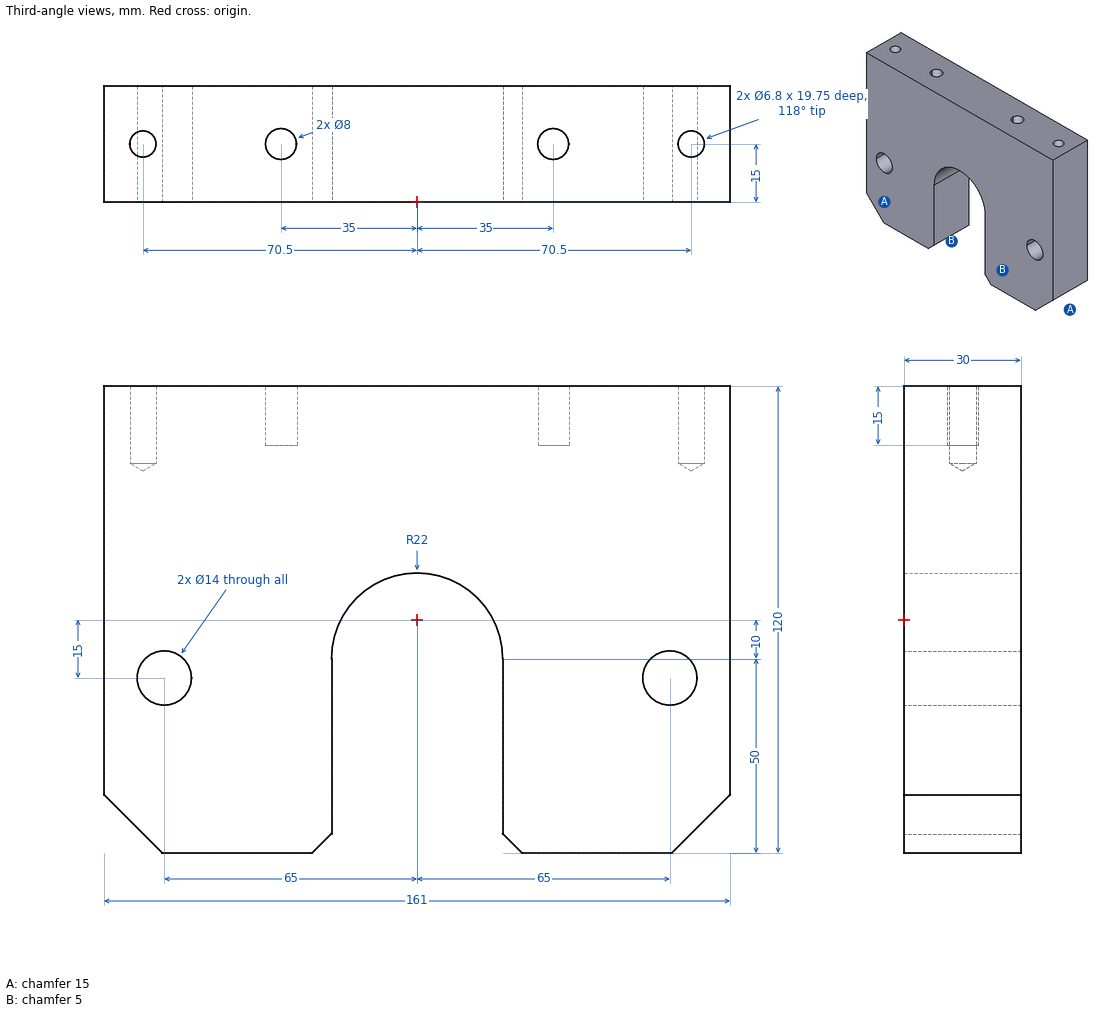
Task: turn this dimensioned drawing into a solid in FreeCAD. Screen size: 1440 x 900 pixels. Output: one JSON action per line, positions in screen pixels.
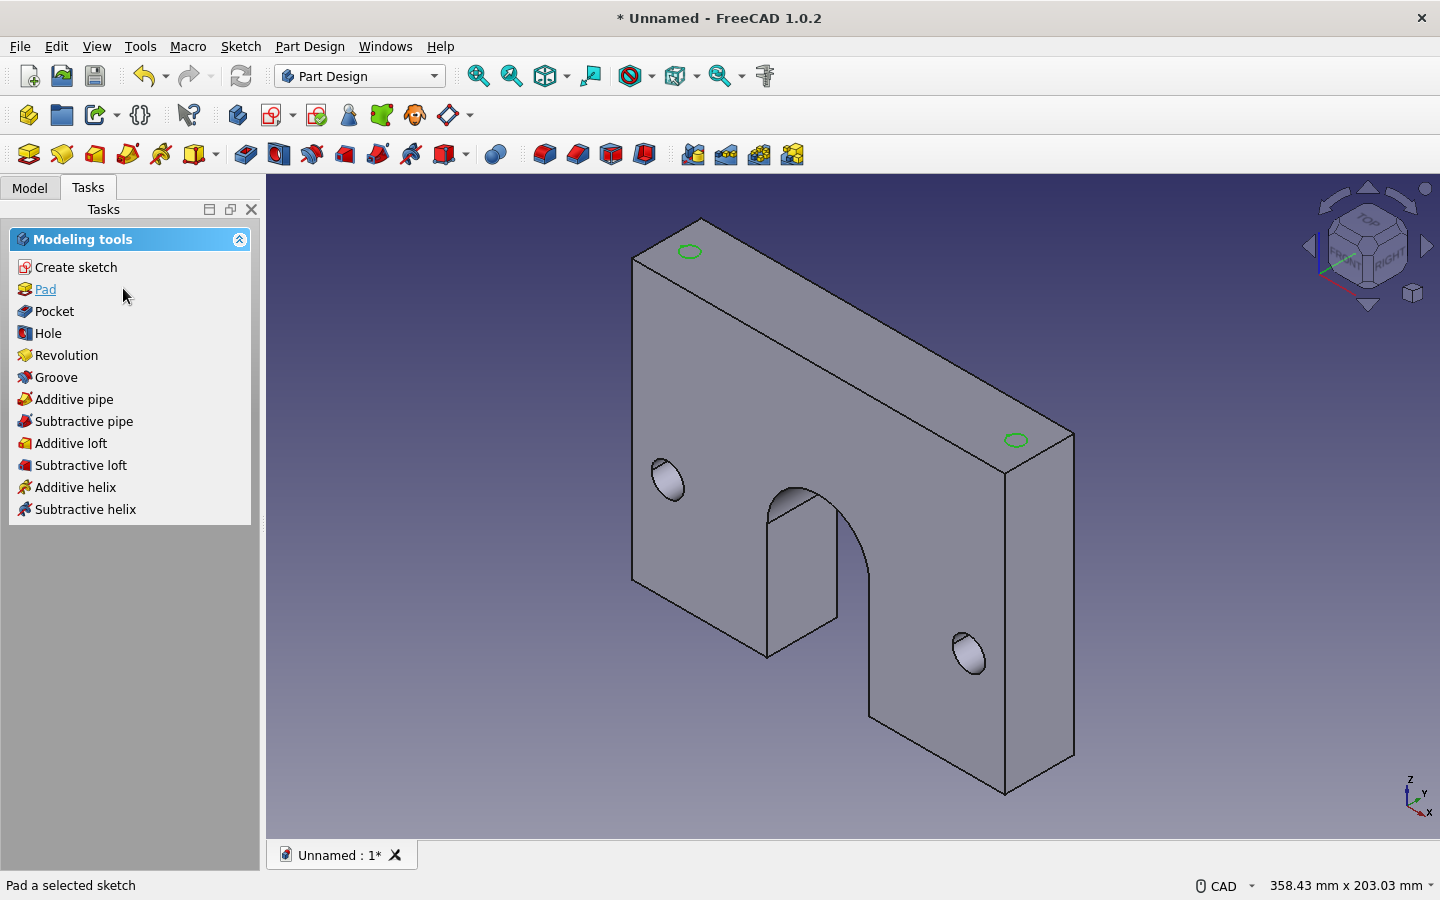
{"action": "left_click", "coordinate": [279, 154]}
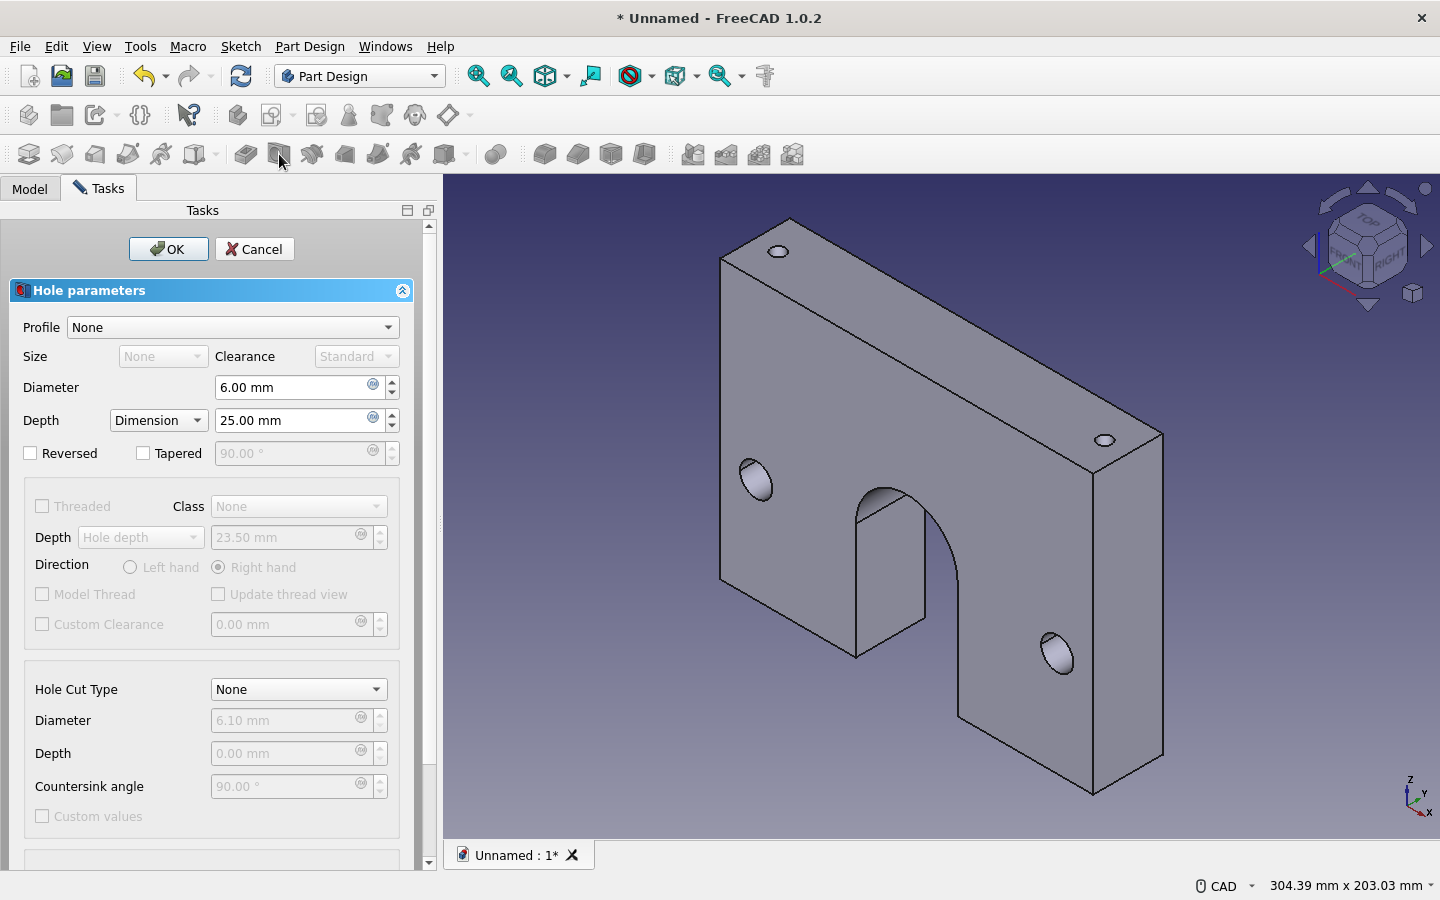
{"action": "triple_click", "coordinate": [300, 388]}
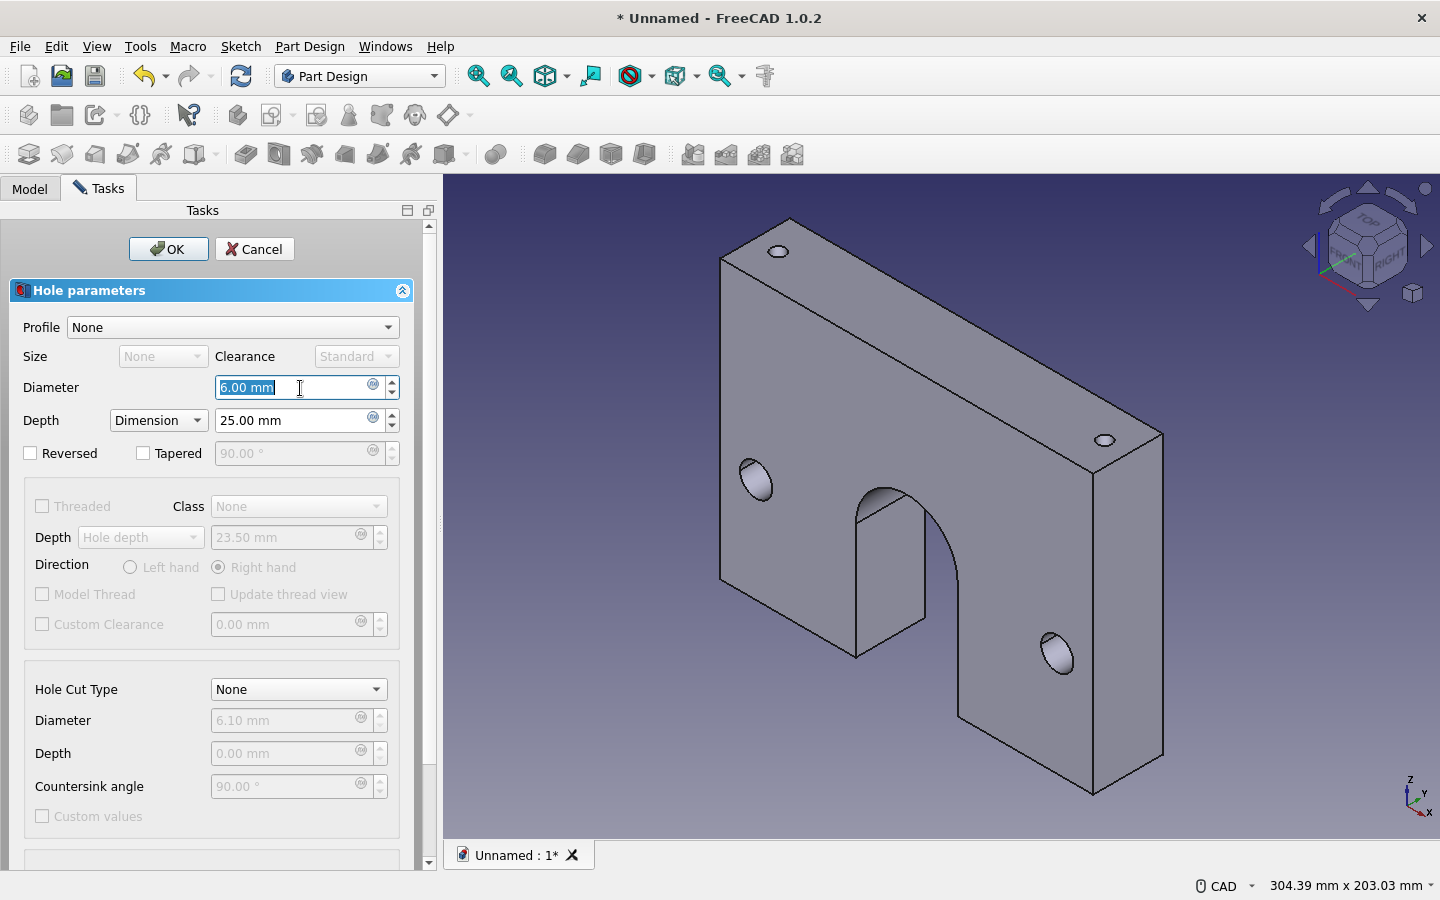
{"action": "type", "text": "6.8"}
{"action": "key", "text": "Tab"}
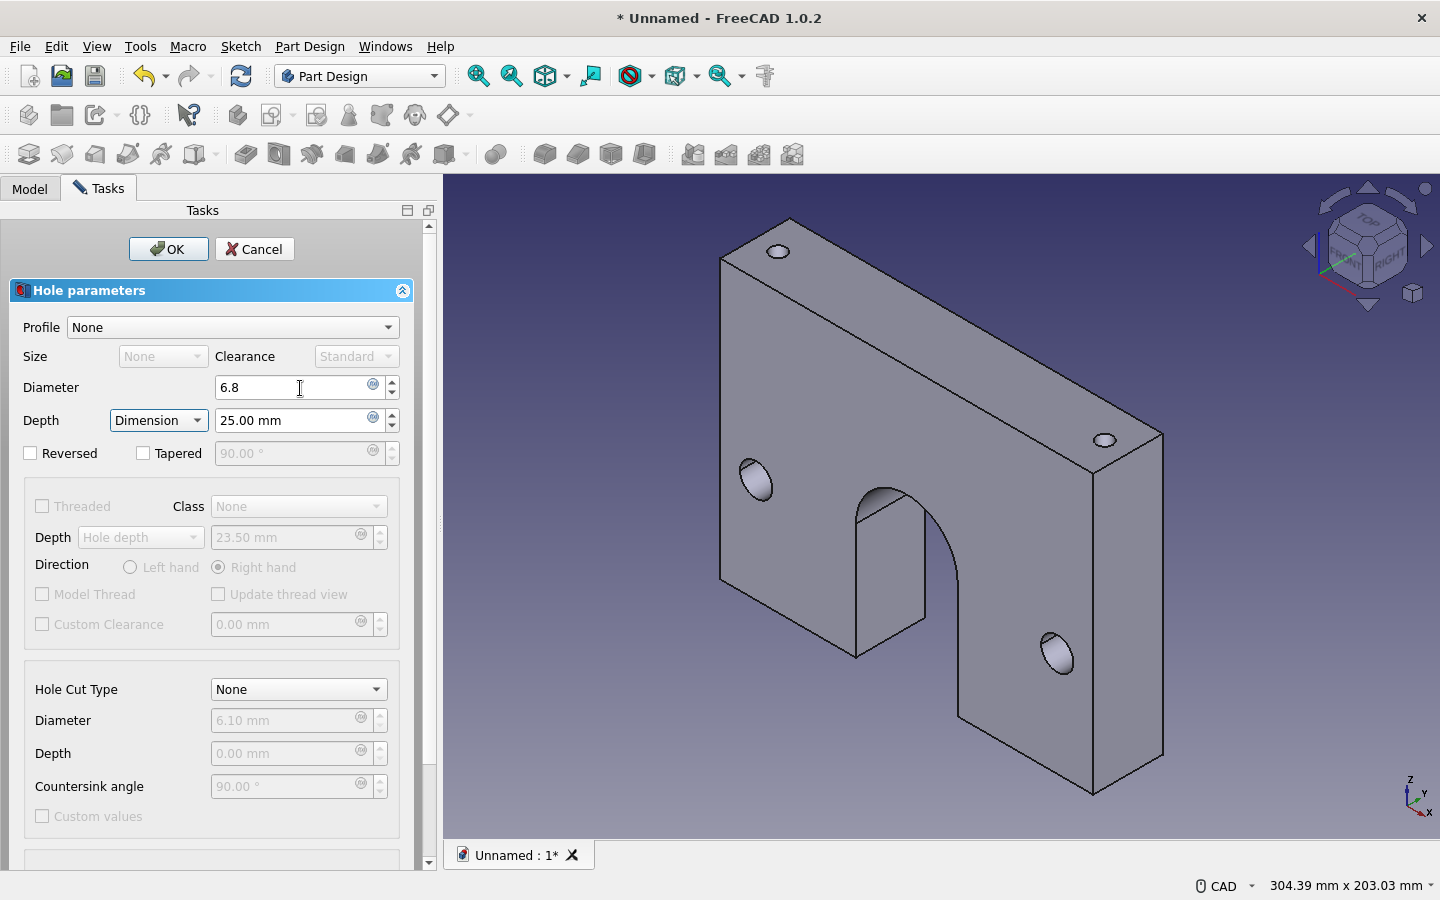
{"action": "triple_click", "coordinate": [300, 420]}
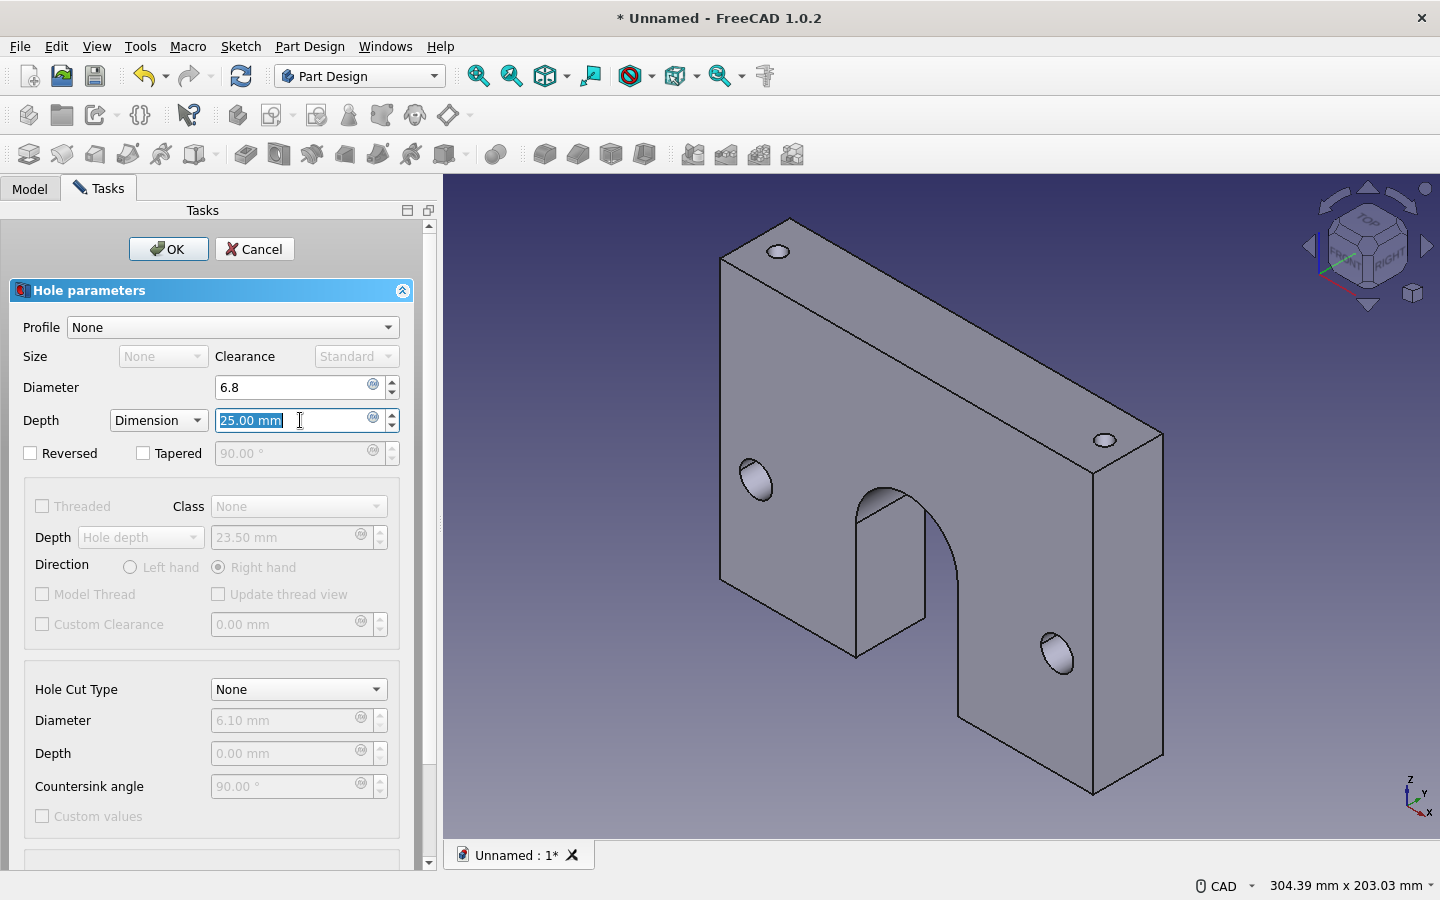
{"action": "type", "text": "19.75"}
{"action": "key", "text": "Tab"}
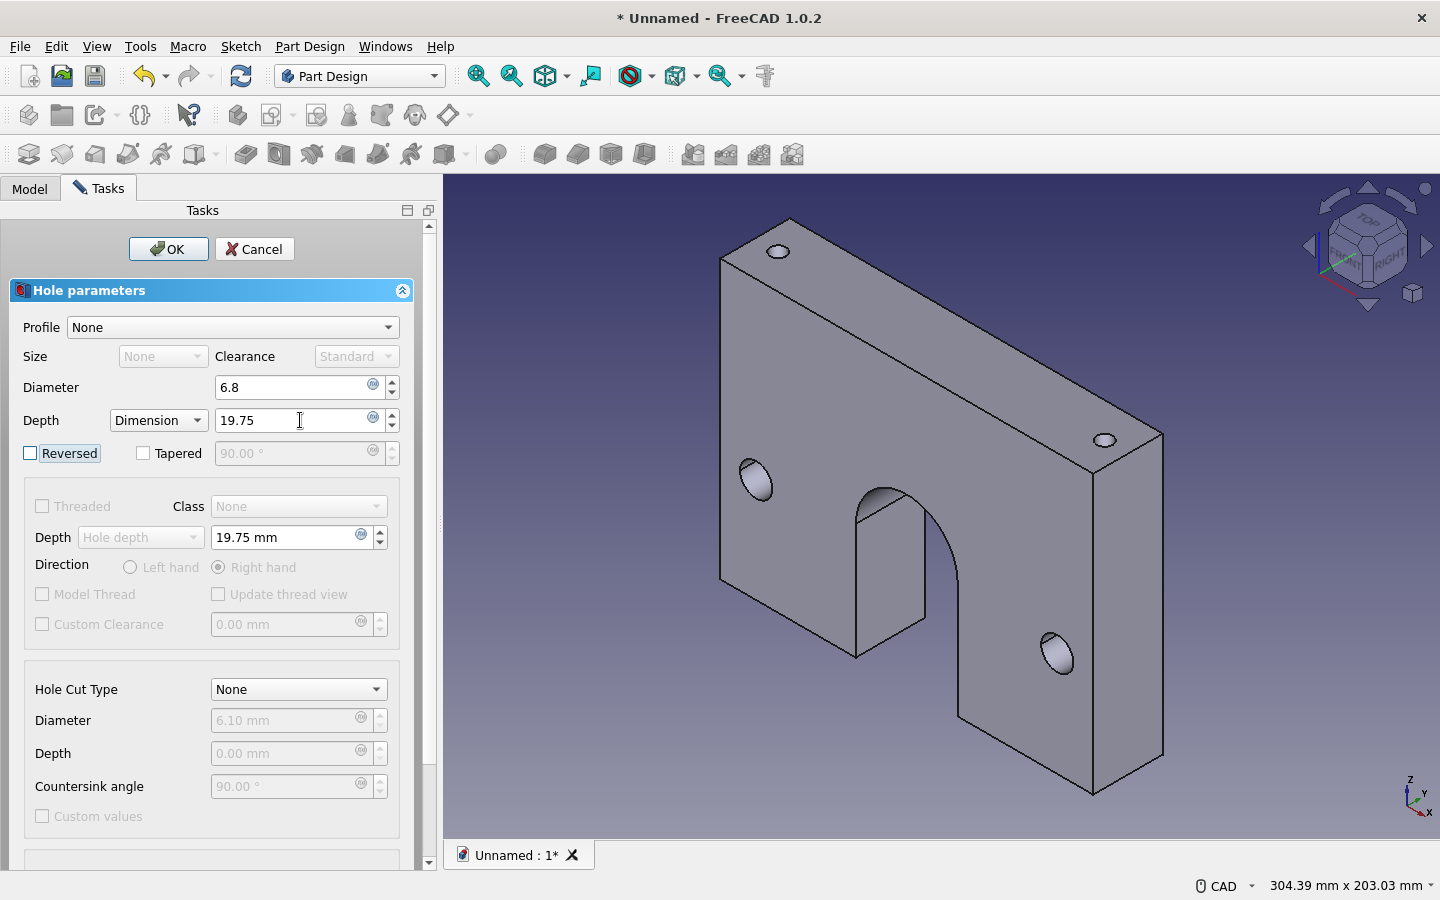
{"action": "left_click", "coordinate": [169, 249]}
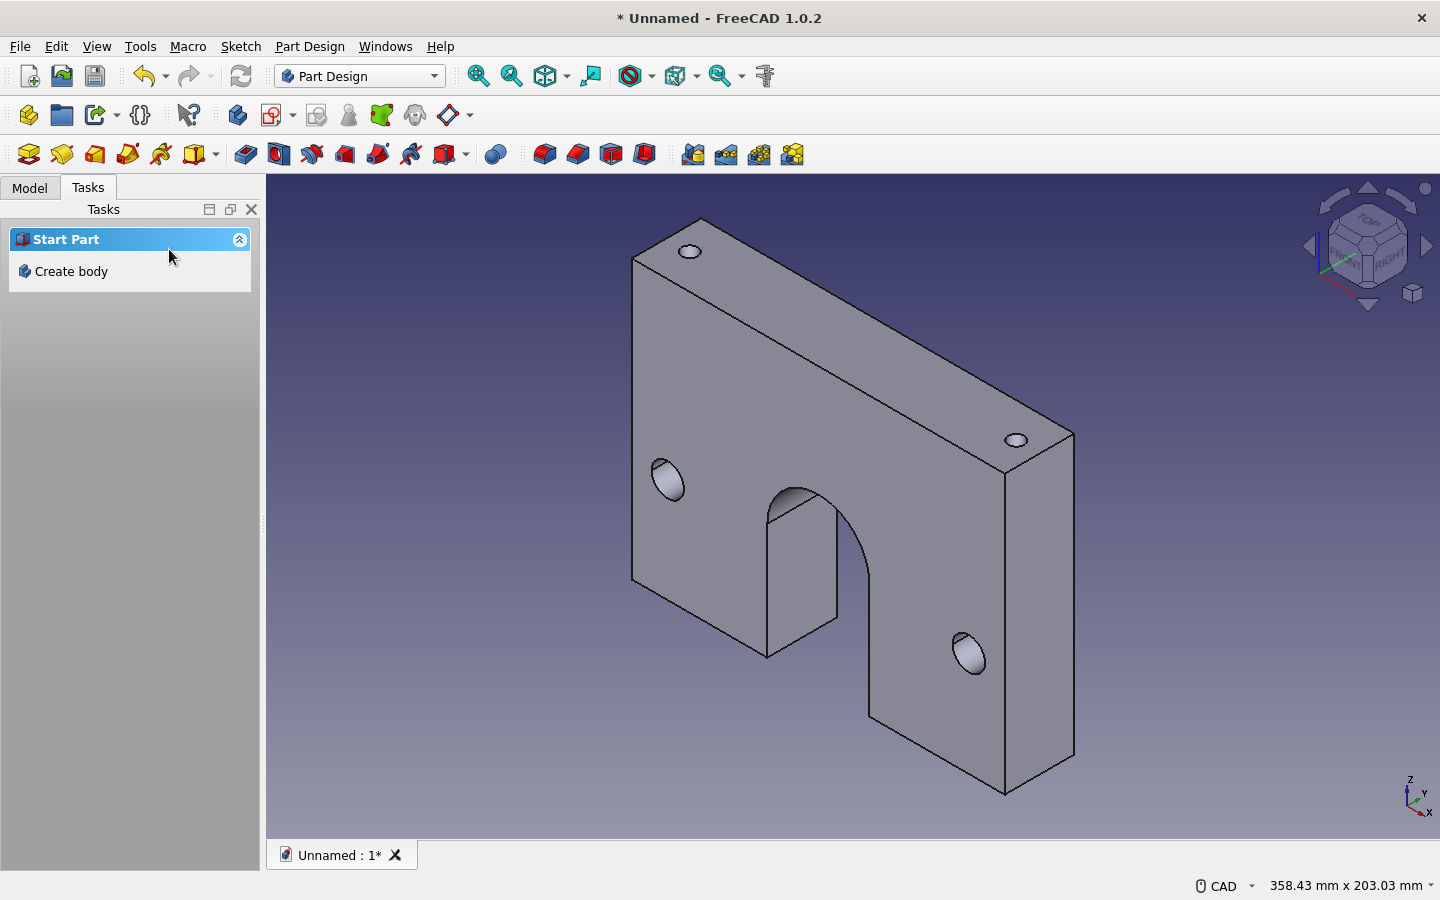
{"action": "left_click", "coordinate": [960, 407]}